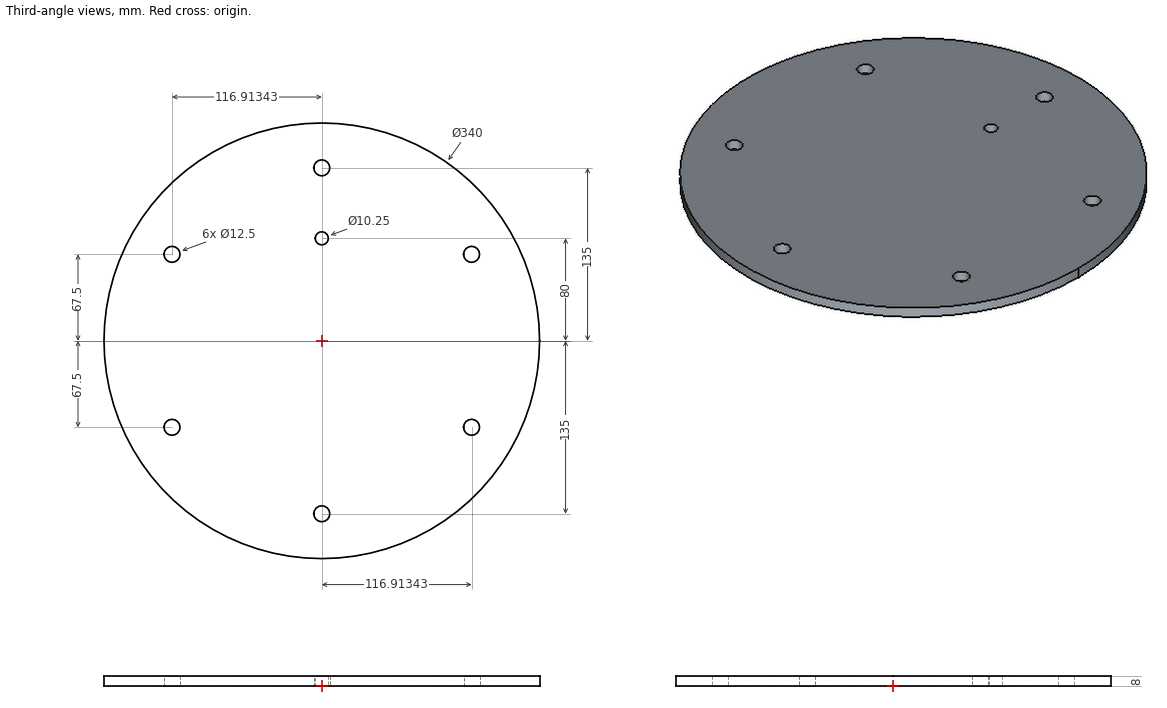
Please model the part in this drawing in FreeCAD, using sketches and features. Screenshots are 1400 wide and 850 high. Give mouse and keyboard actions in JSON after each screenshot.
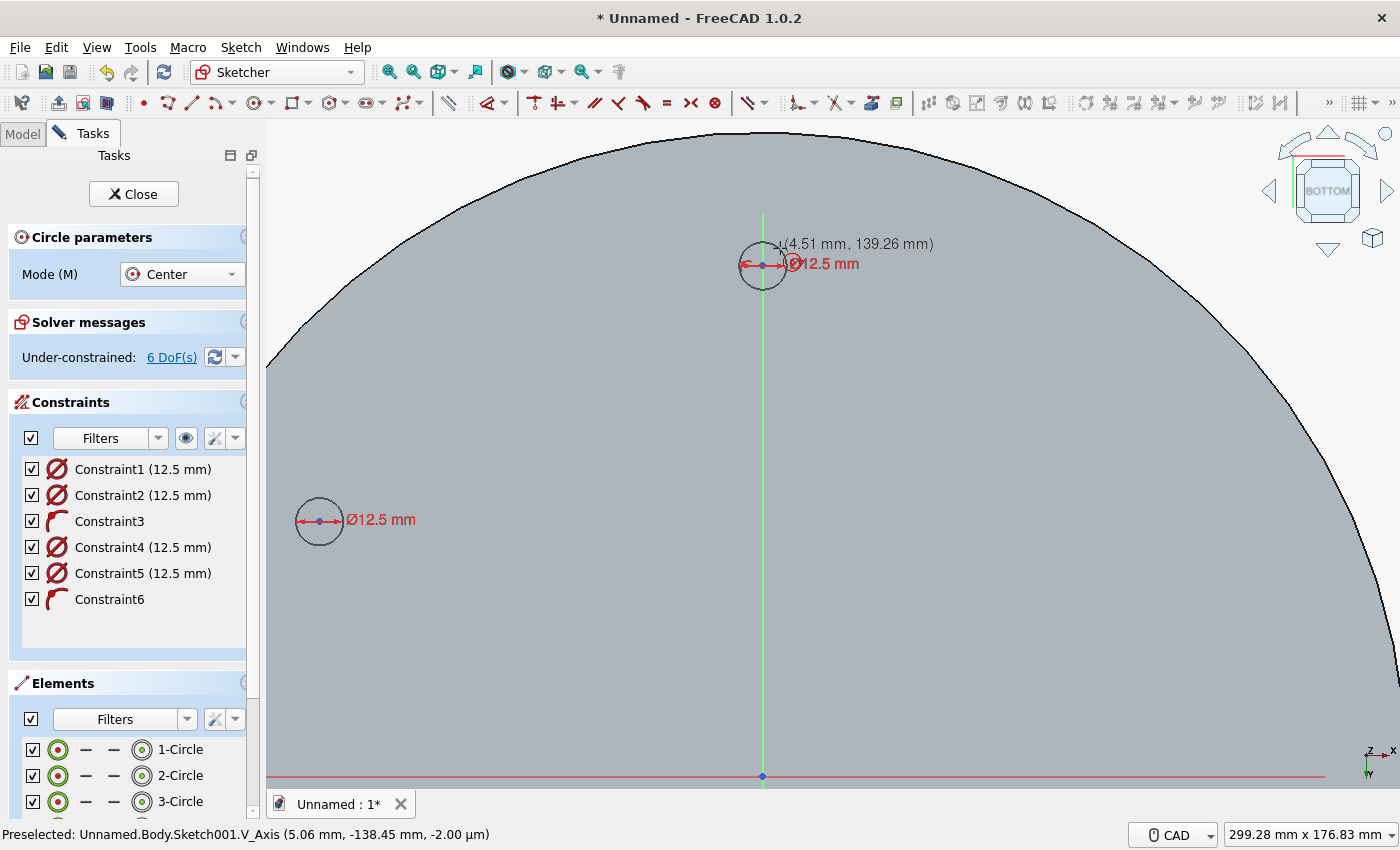
{"action": "left_click", "coordinate": [1206, 521]}
{"action": "mouse_move", "coordinate": [1223, 504]}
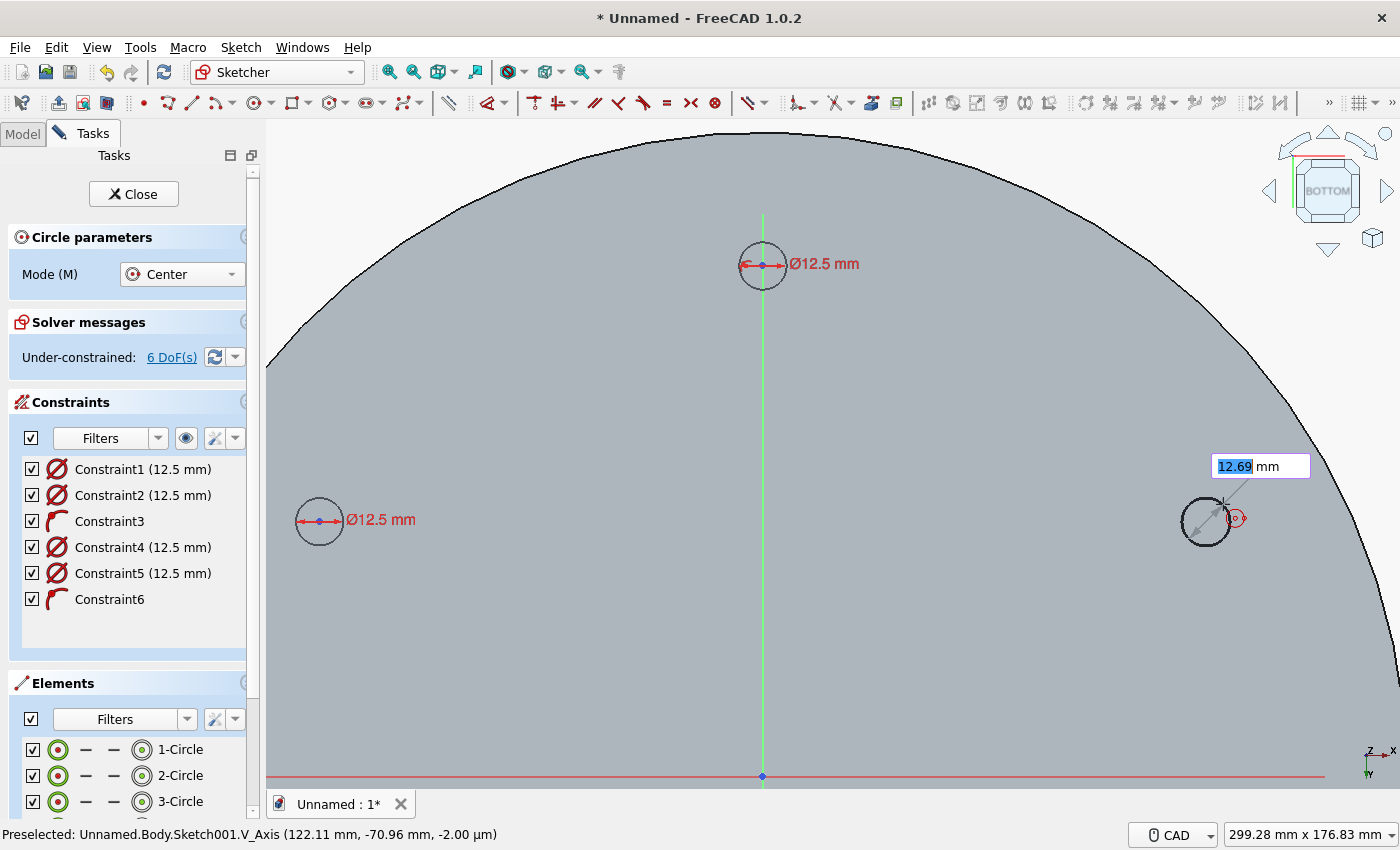
{"action": "type", "text": "12.5"}
{"action": "key", "text": "Return"}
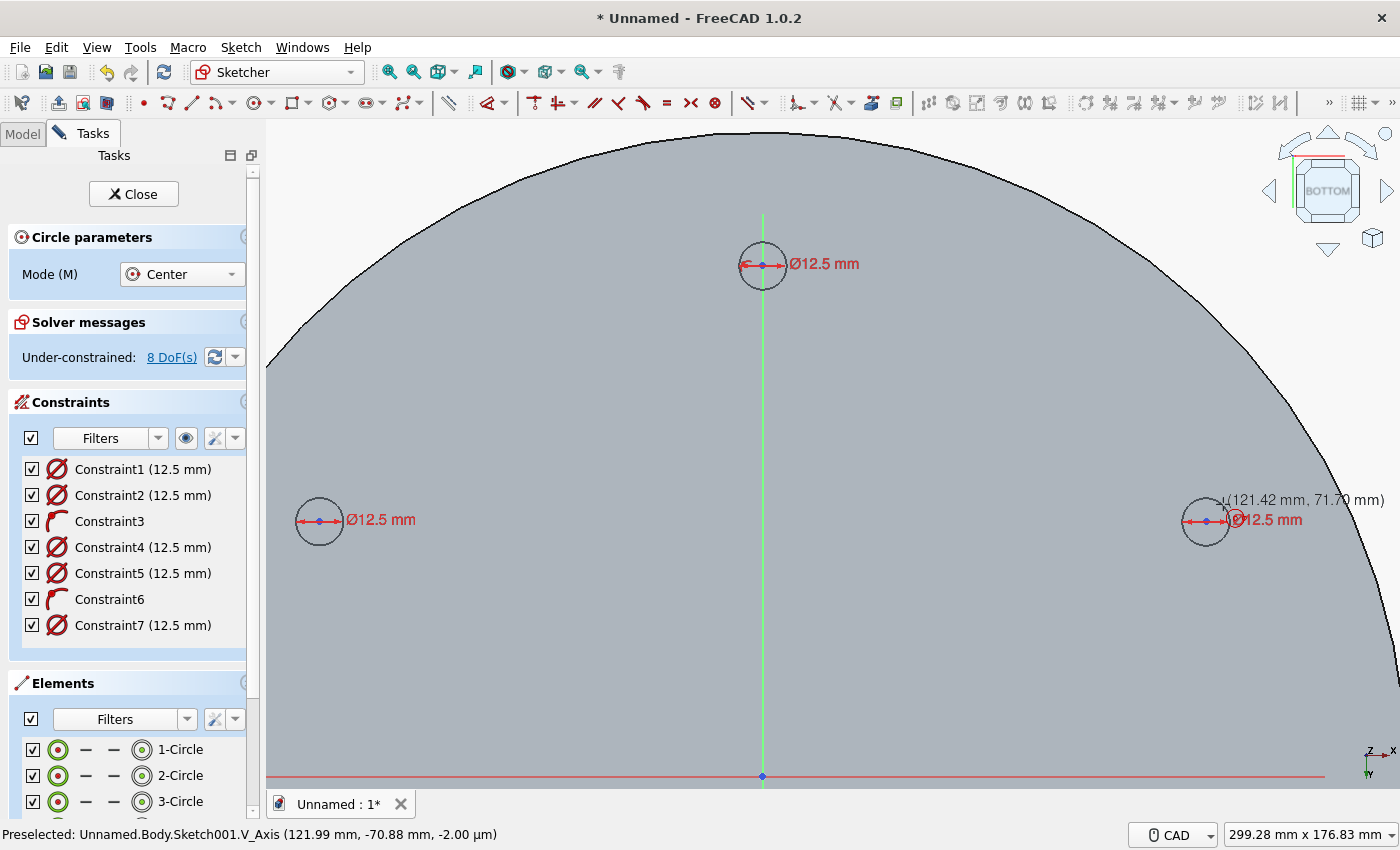
{"action": "scroll", "coordinate": [765, 266], "scroll_direction": "down", "scroll_amount": 5}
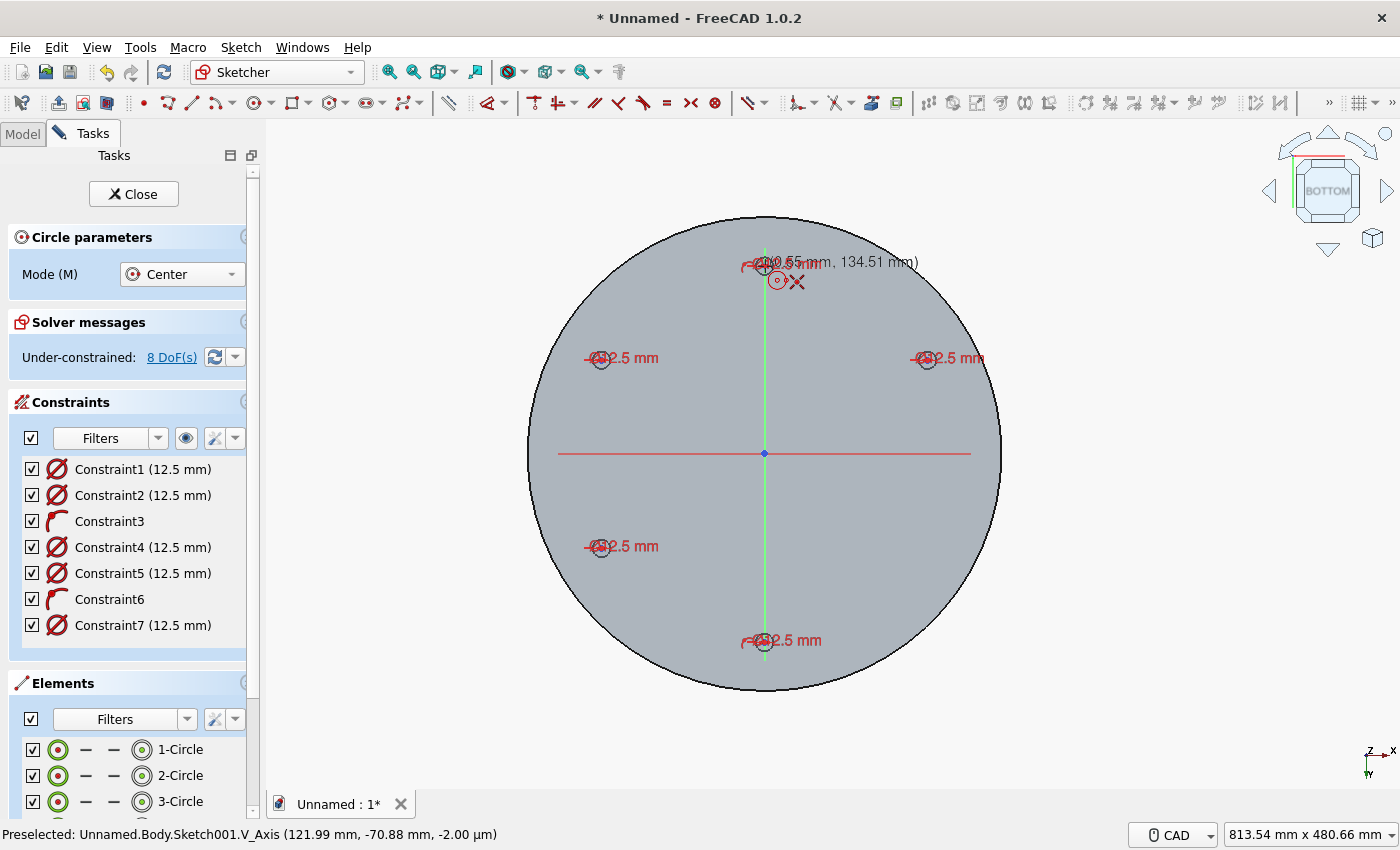
{"action": "scroll", "coordinate": [927, 548], "scroll_direction": "up", "scroll_amount": 5}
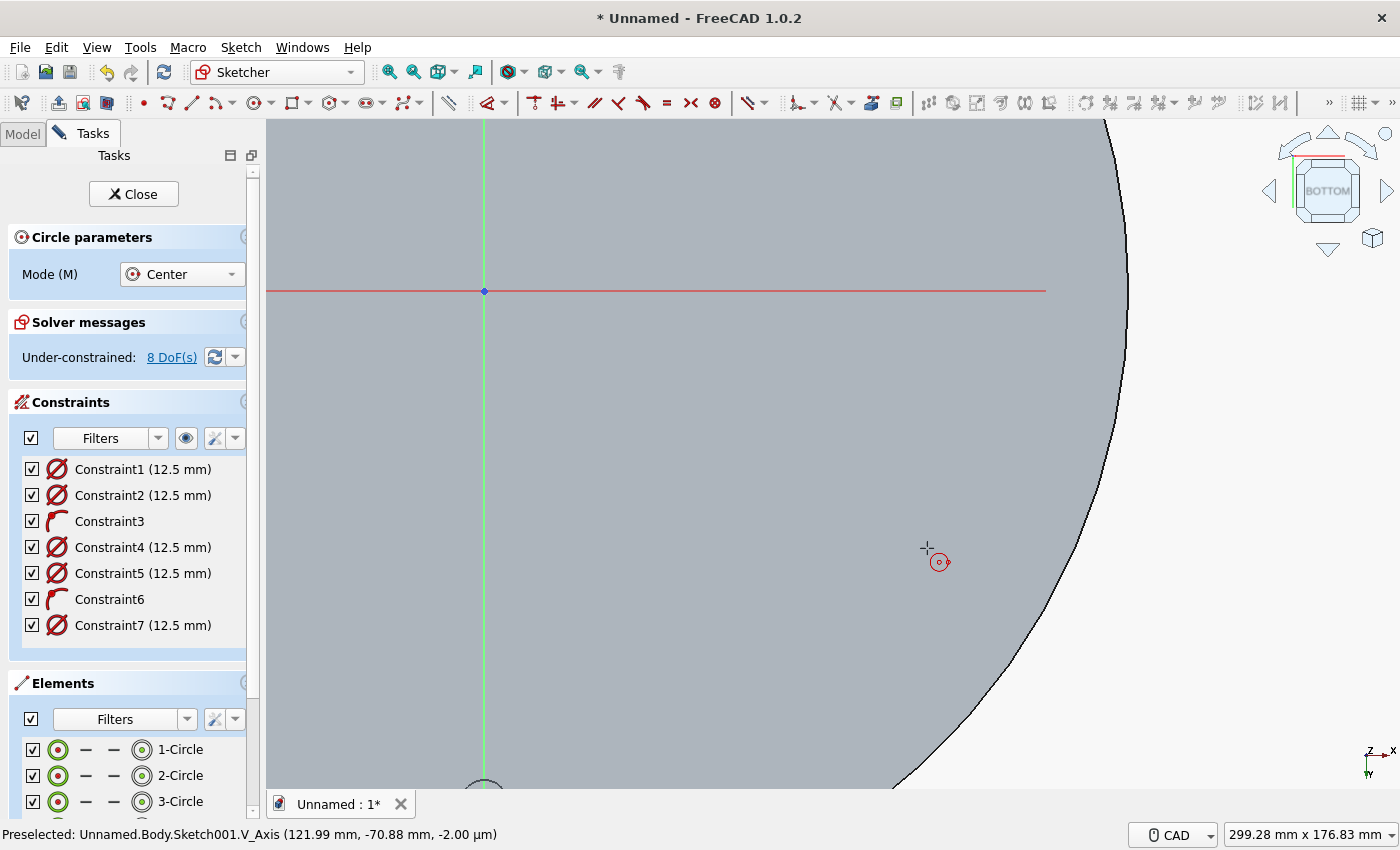
{"action": "left_click", "coordinate": [927, 547]}
{"action": "mouse_move", "coordinate": [944, 530]}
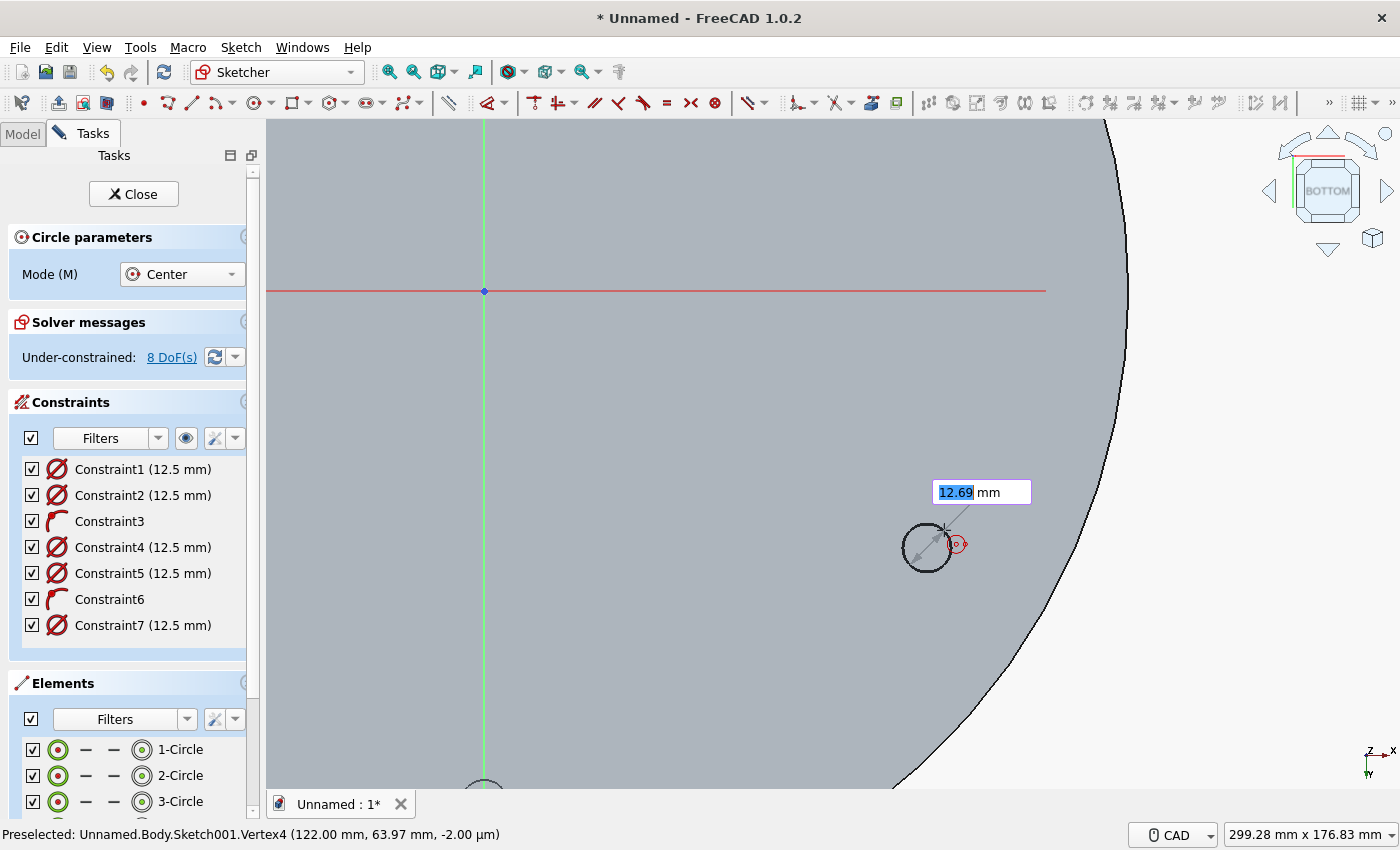
{"action": "type", "text": "12.5"}
{"action": "key", "text": "Return"}
{"action": "key", "text": "Escape"}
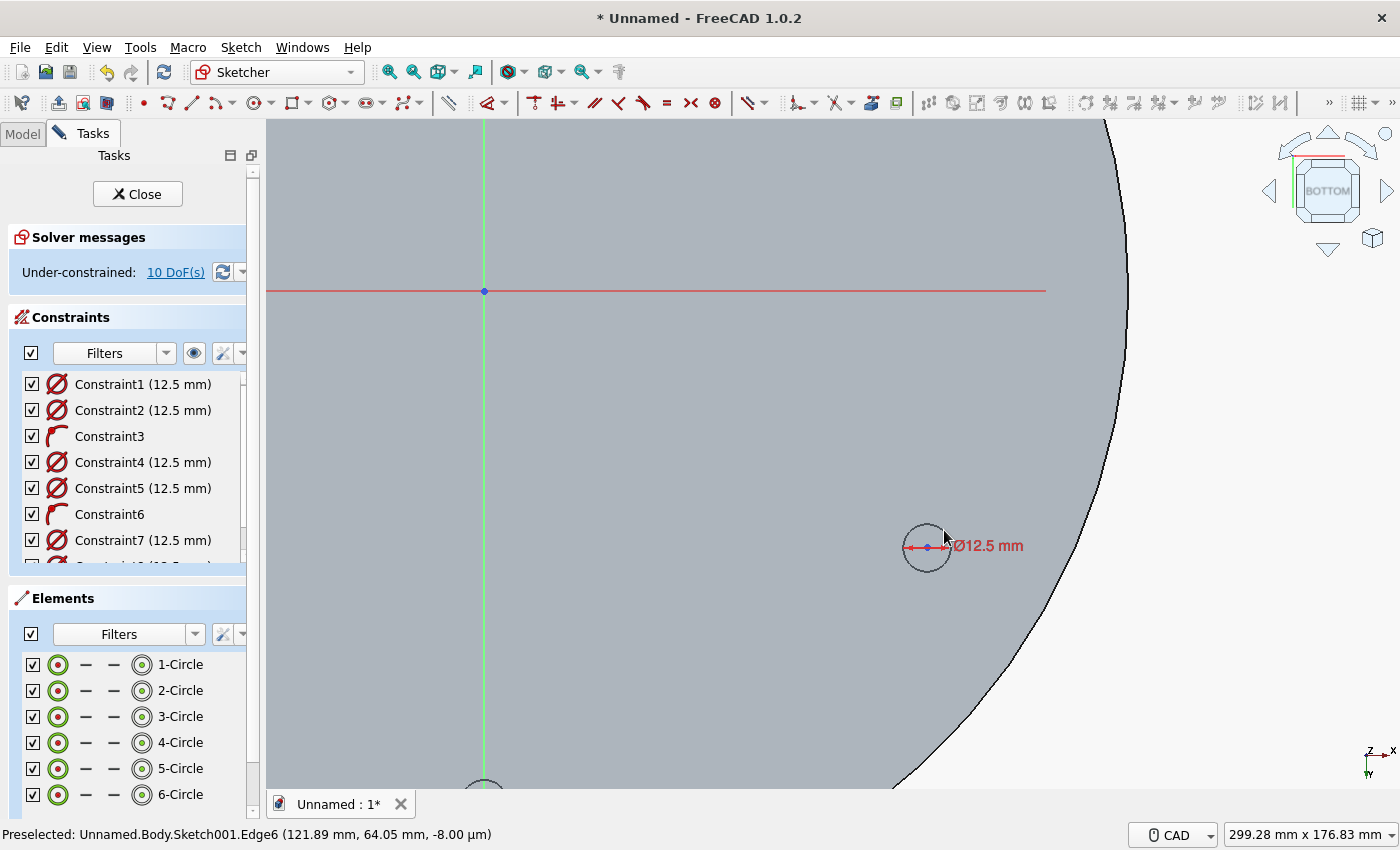
{"action": "scroll", "coordinate": [928, 549], "scroll_direction": "down", "scroll_amount": 5}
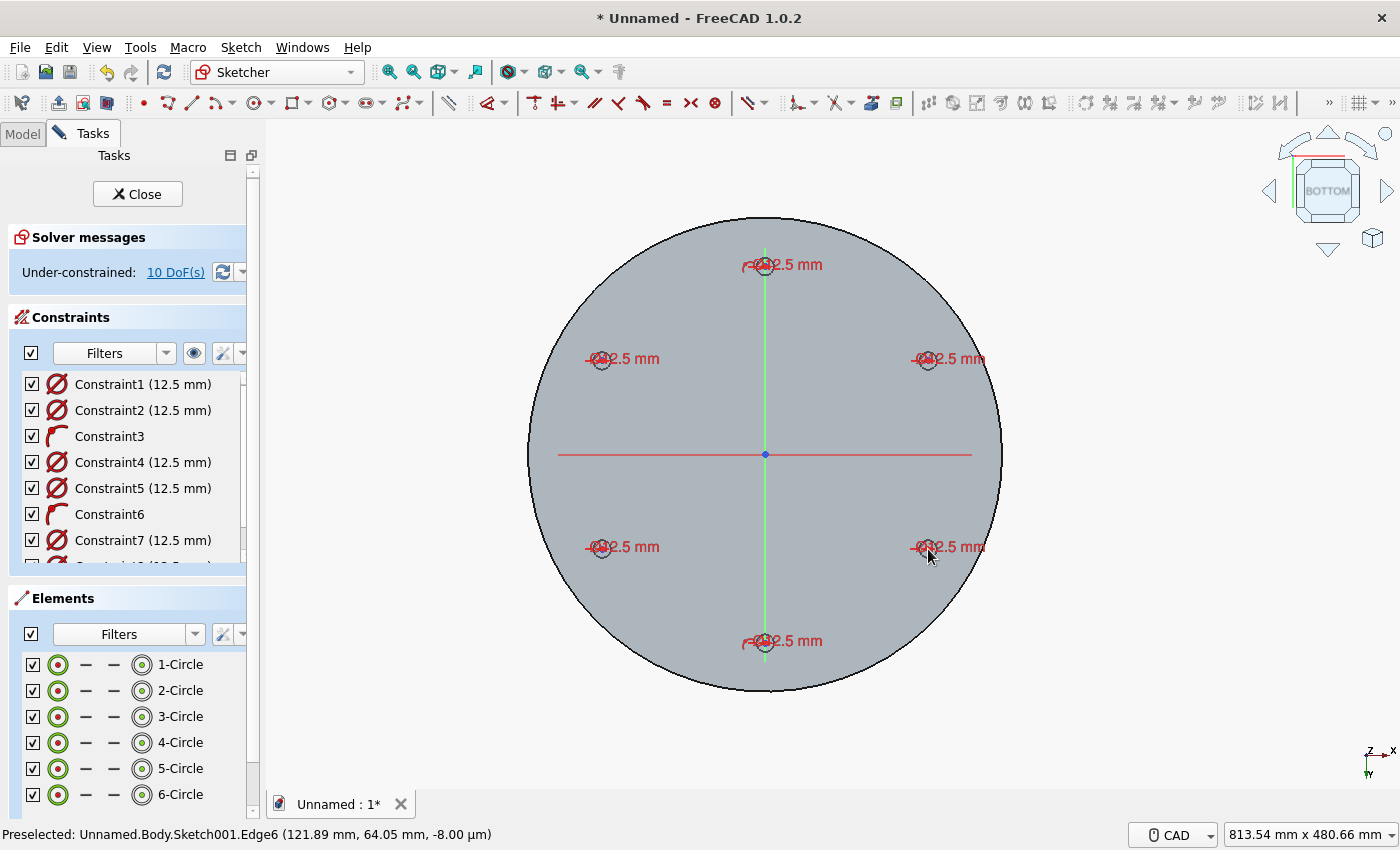
{"action": "left_click", "coordinate": [602, 549]}